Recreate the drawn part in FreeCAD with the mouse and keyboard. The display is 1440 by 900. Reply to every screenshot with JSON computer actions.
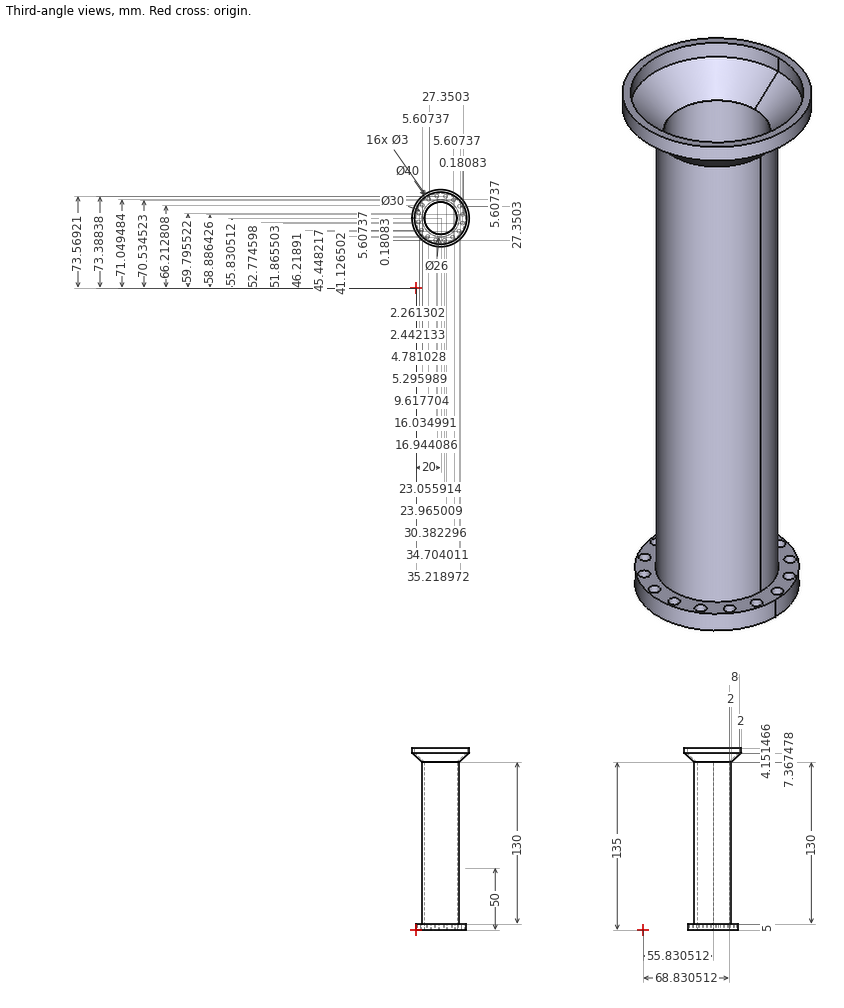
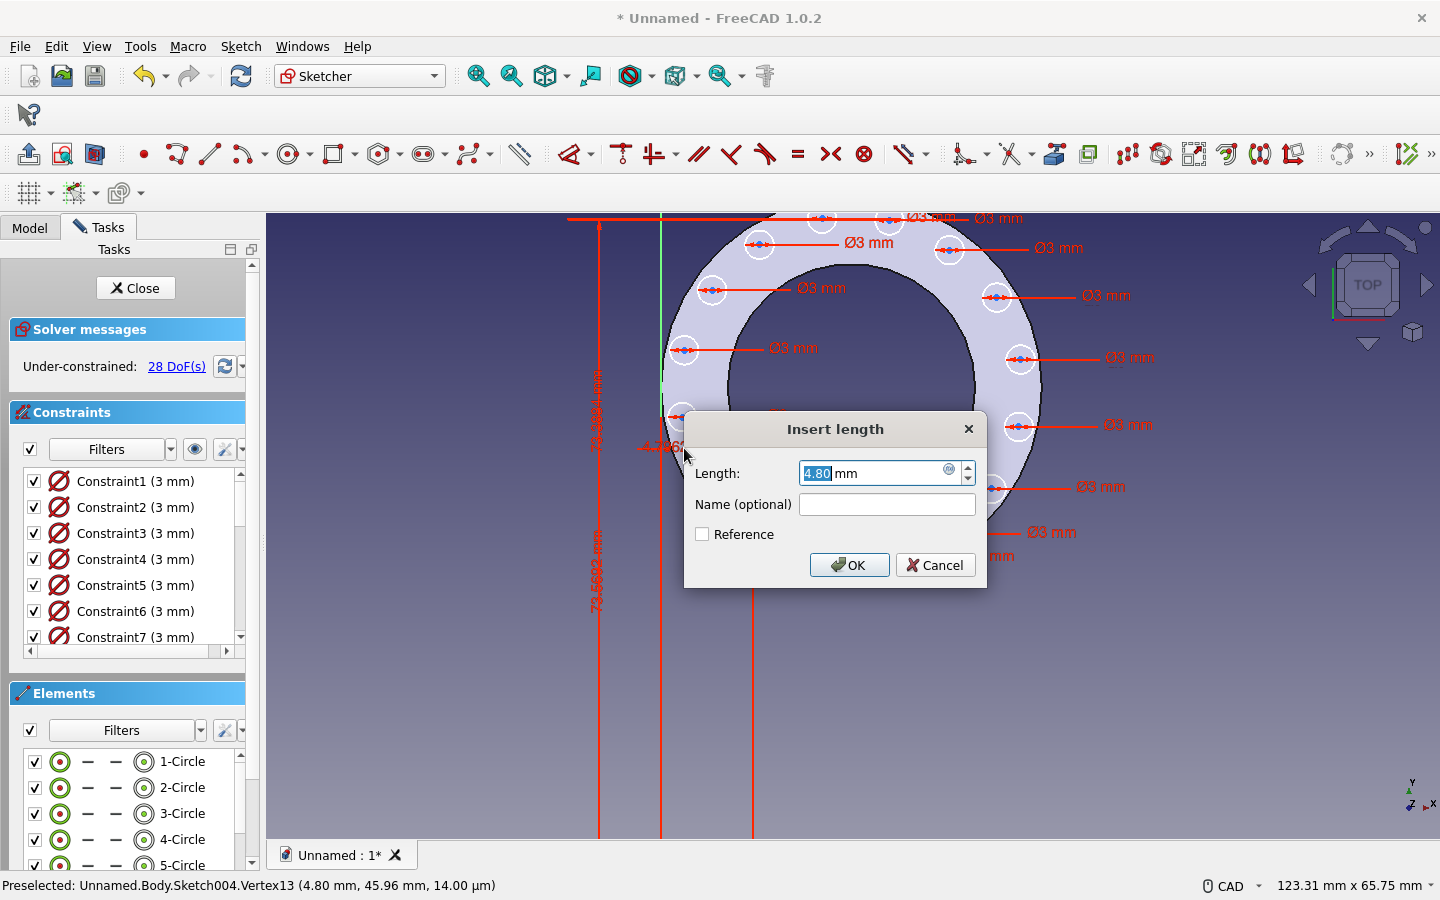
{"action": "type", "text": "4.781028"}
{"action": "key", "text": "Return"}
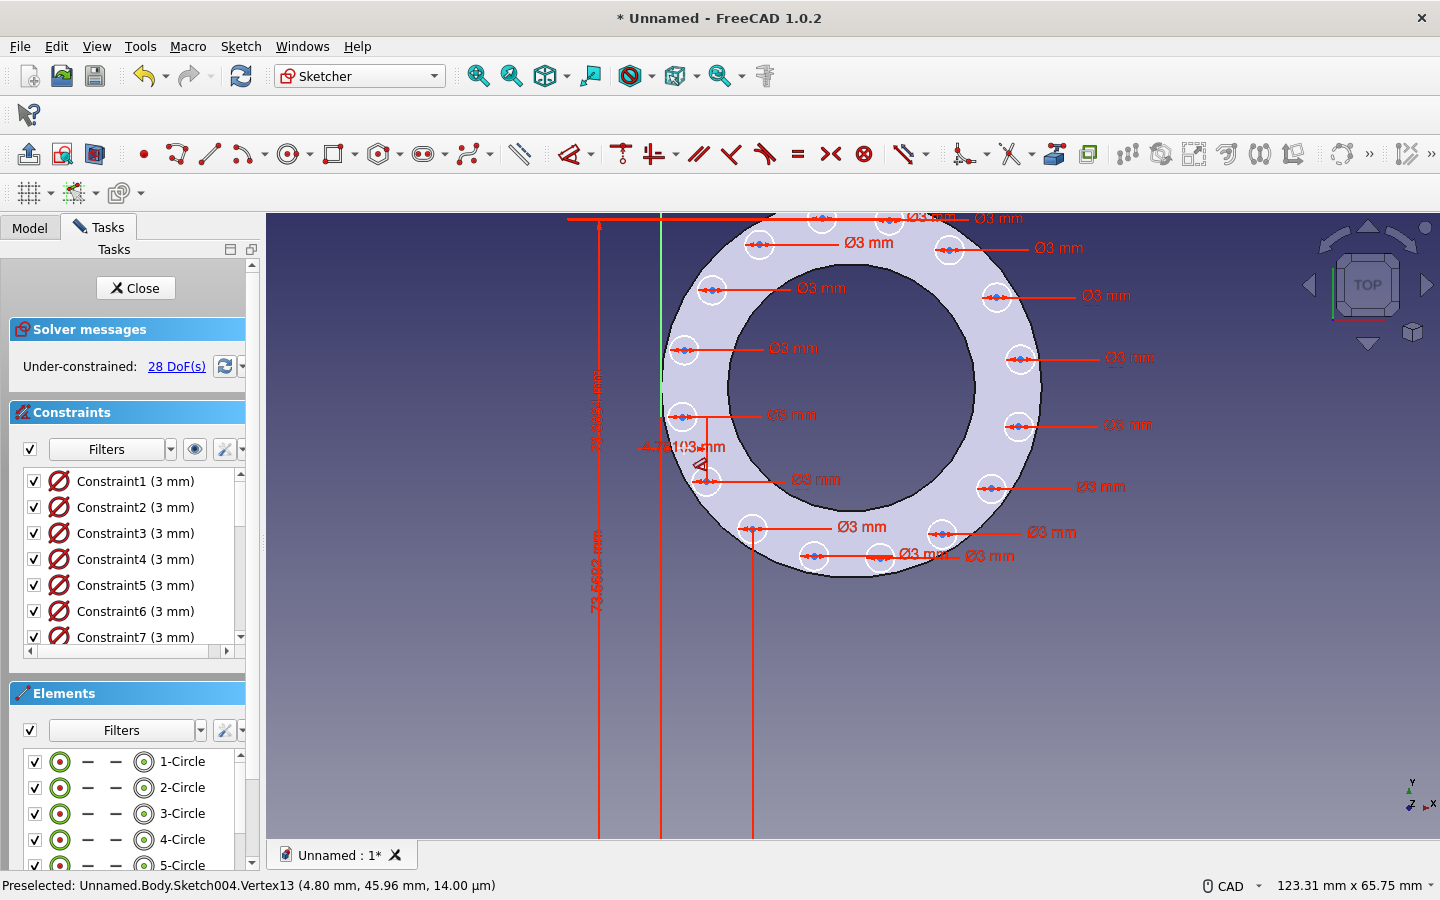
{"action": "left_click", "coordinate": [707, 482]}
{"action": "left_click", "coordinate": [627, 646]}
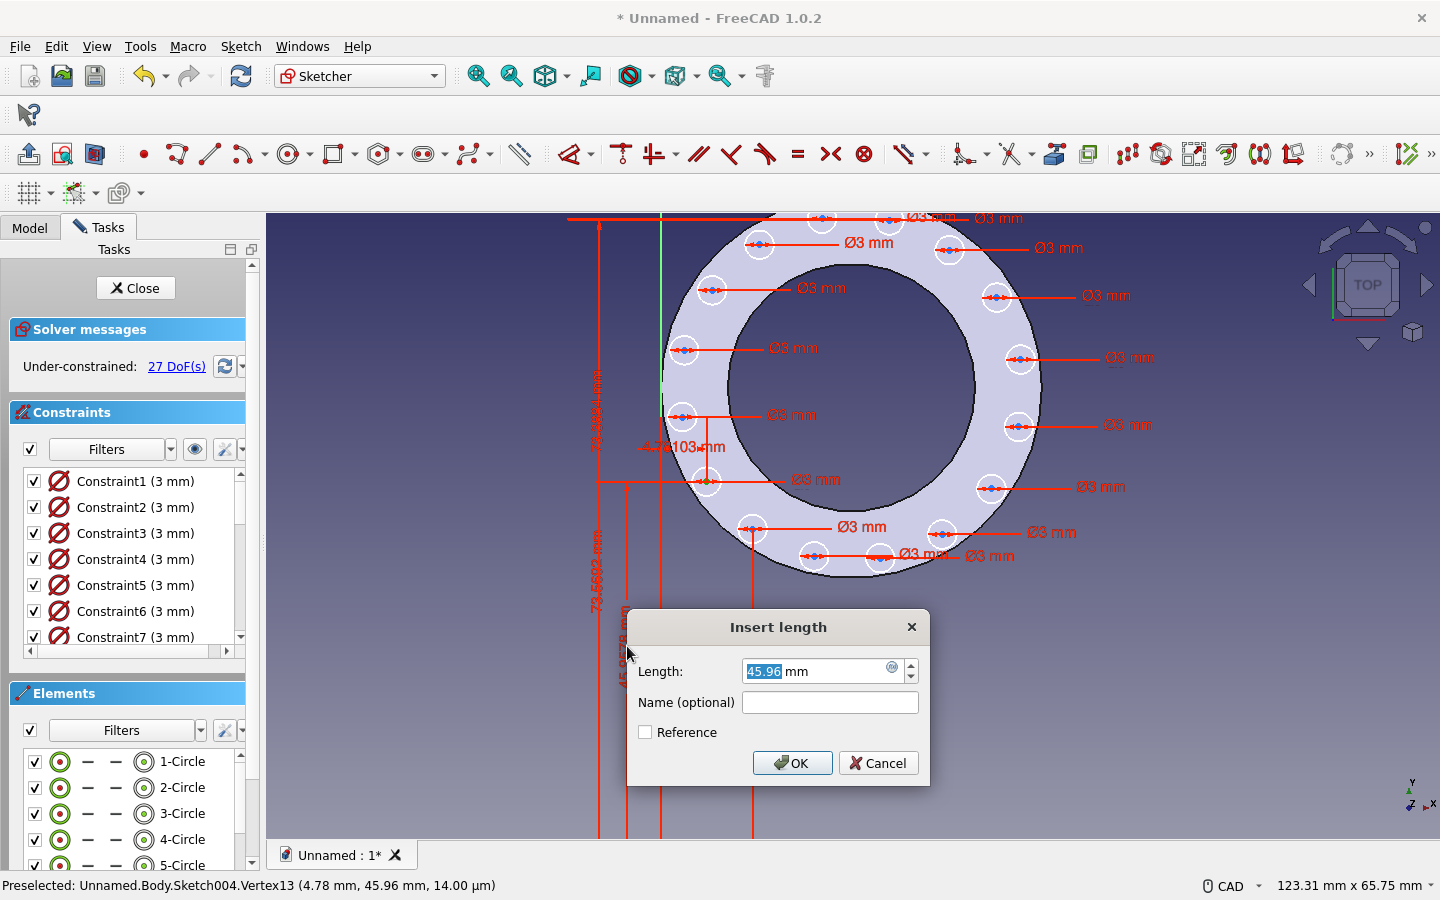
{"action": "type", "text": "46.21891"}
{"action": "key", "text": "Return"}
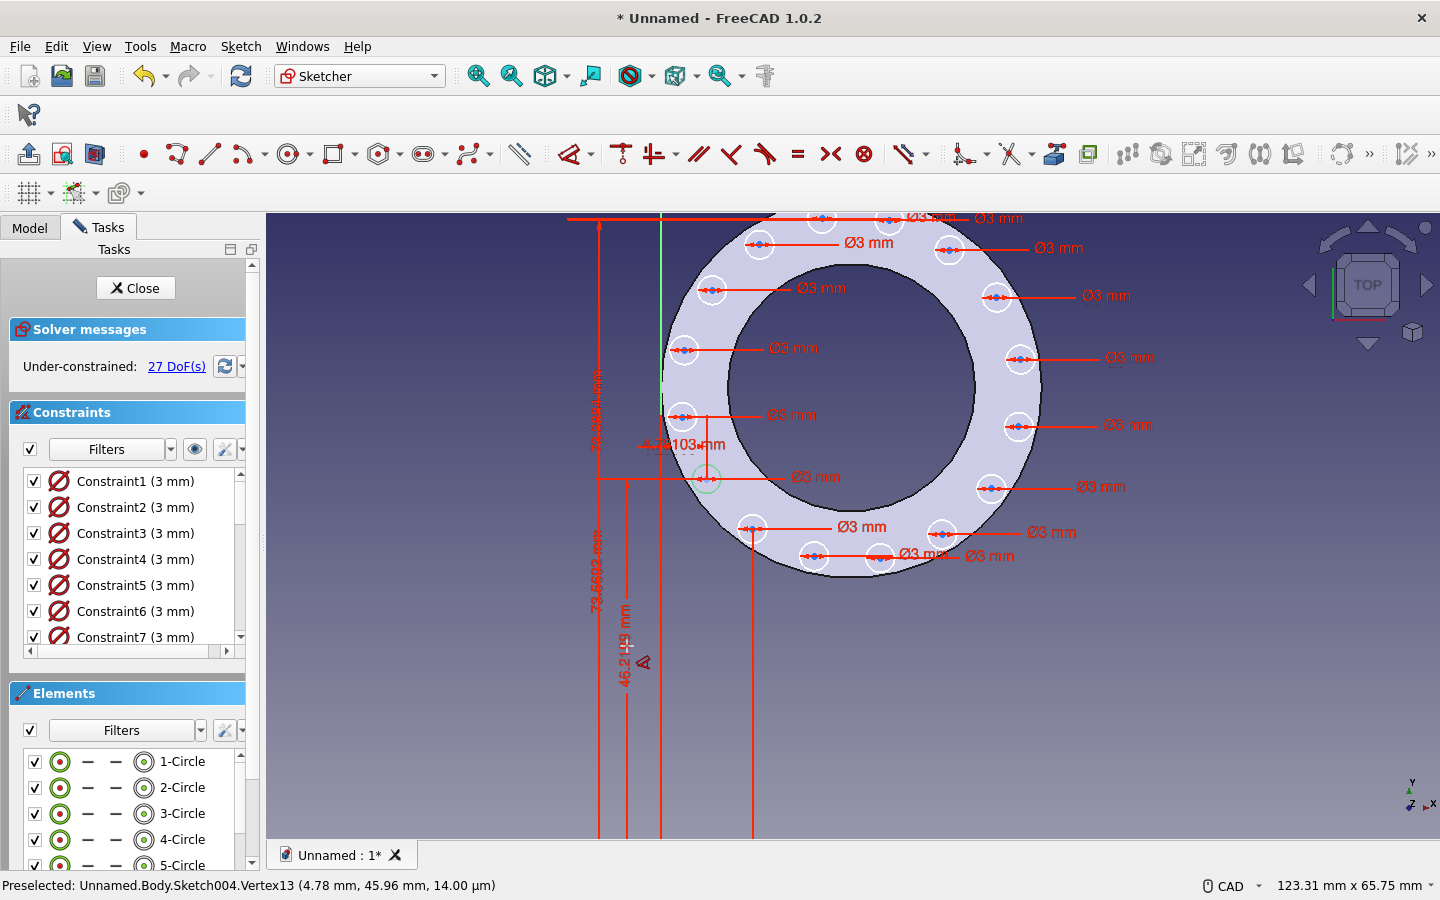
{"action": "scroll", "coordinate": [682, 417], "scroll_direction": "up", "scroll_amount": 4}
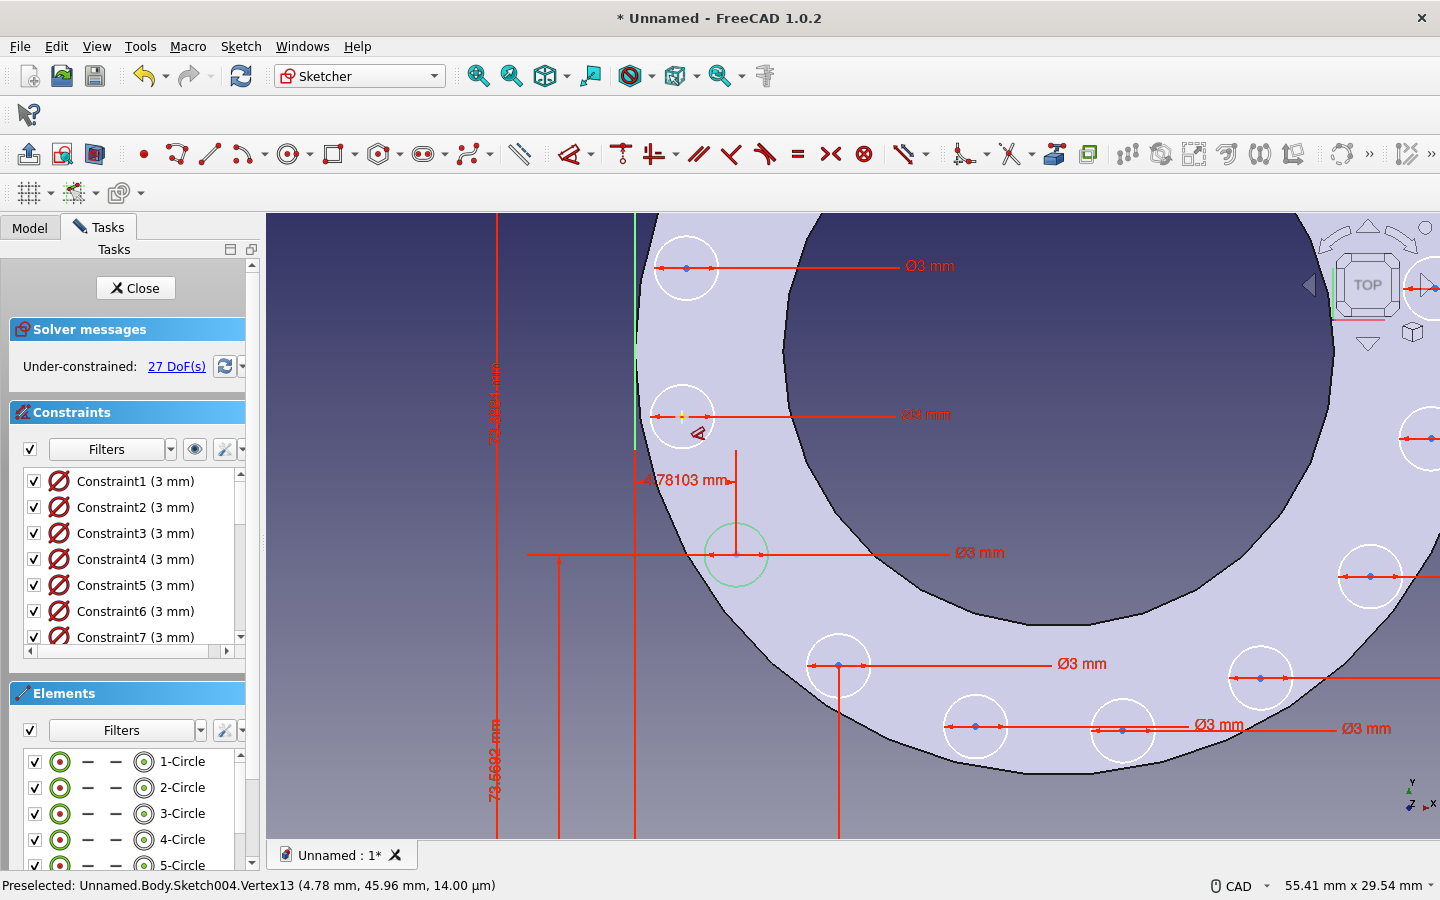
{"action": "left_click", "coordinate": [682, 417]}
{"action": "left_click", "coordinate": [659, 359]}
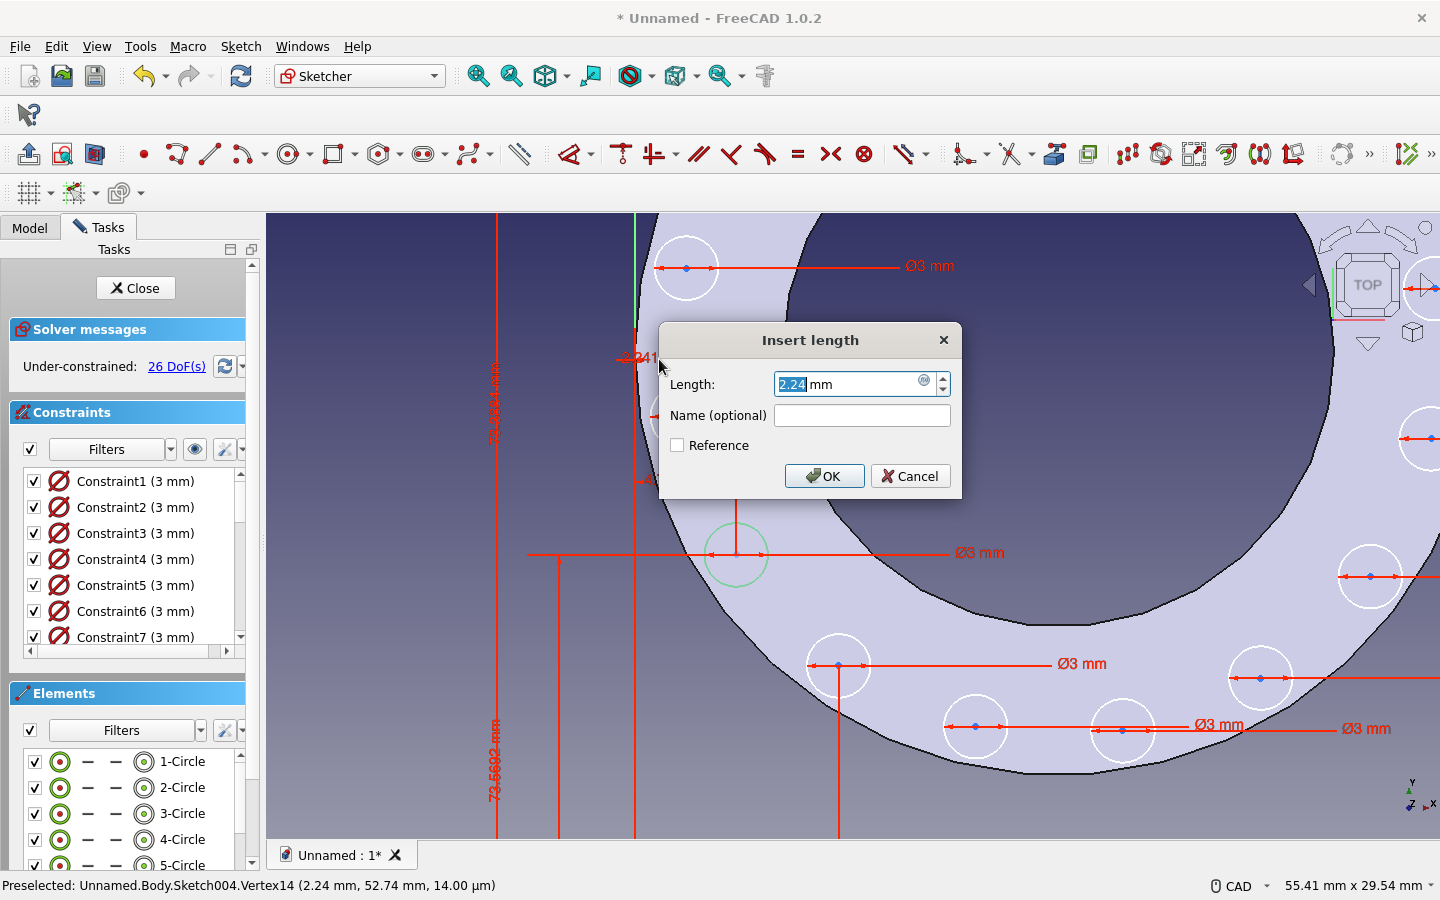
{"action": "type", "text": "2.261302"}
{"action": "key", "text": "Return"}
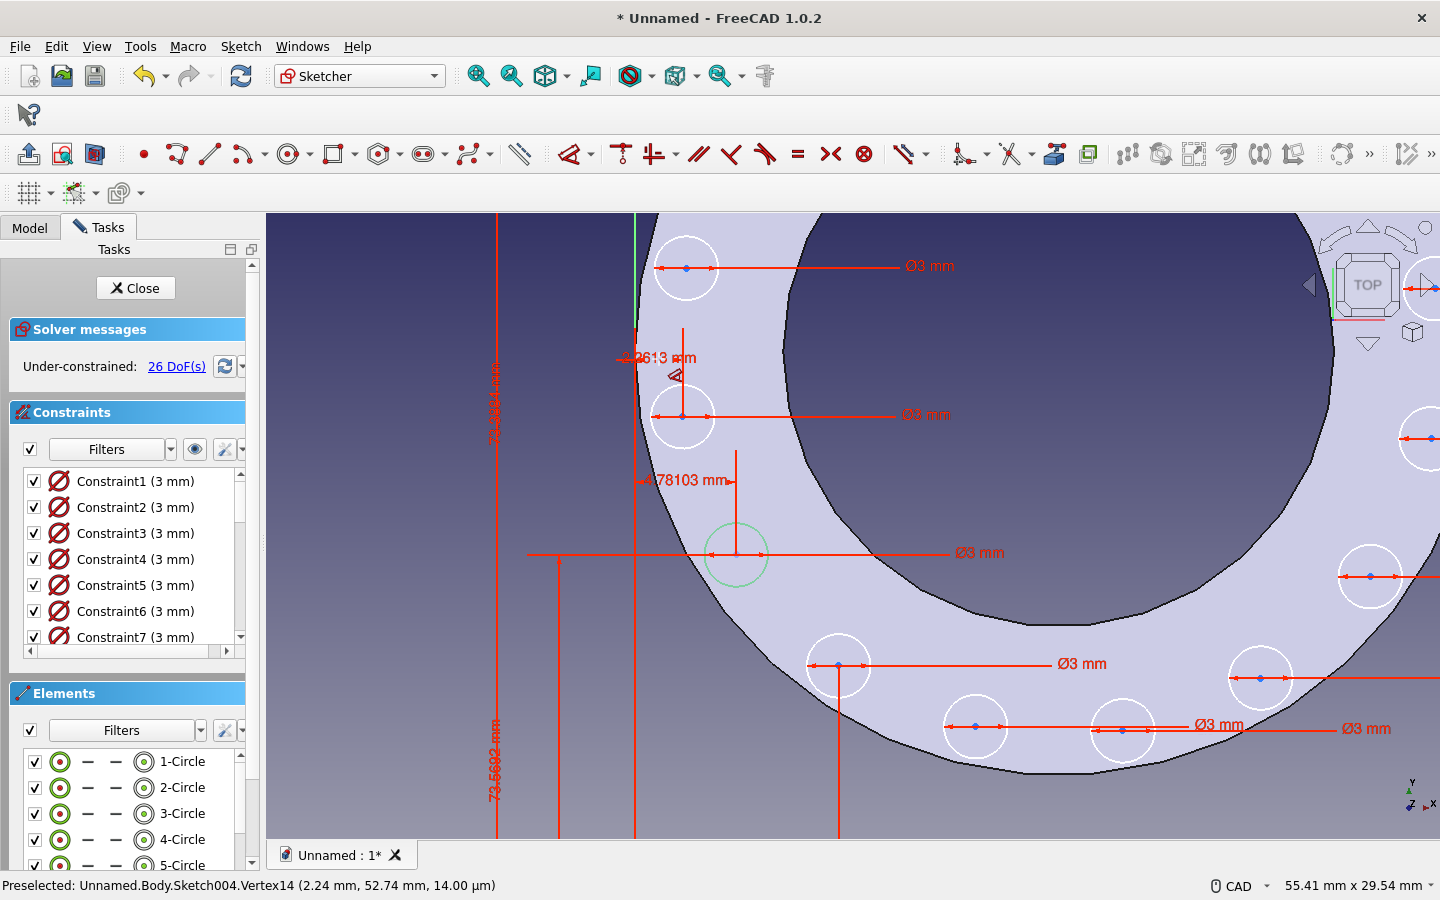
{"action": "left_click", "coordinate": [686, 268]}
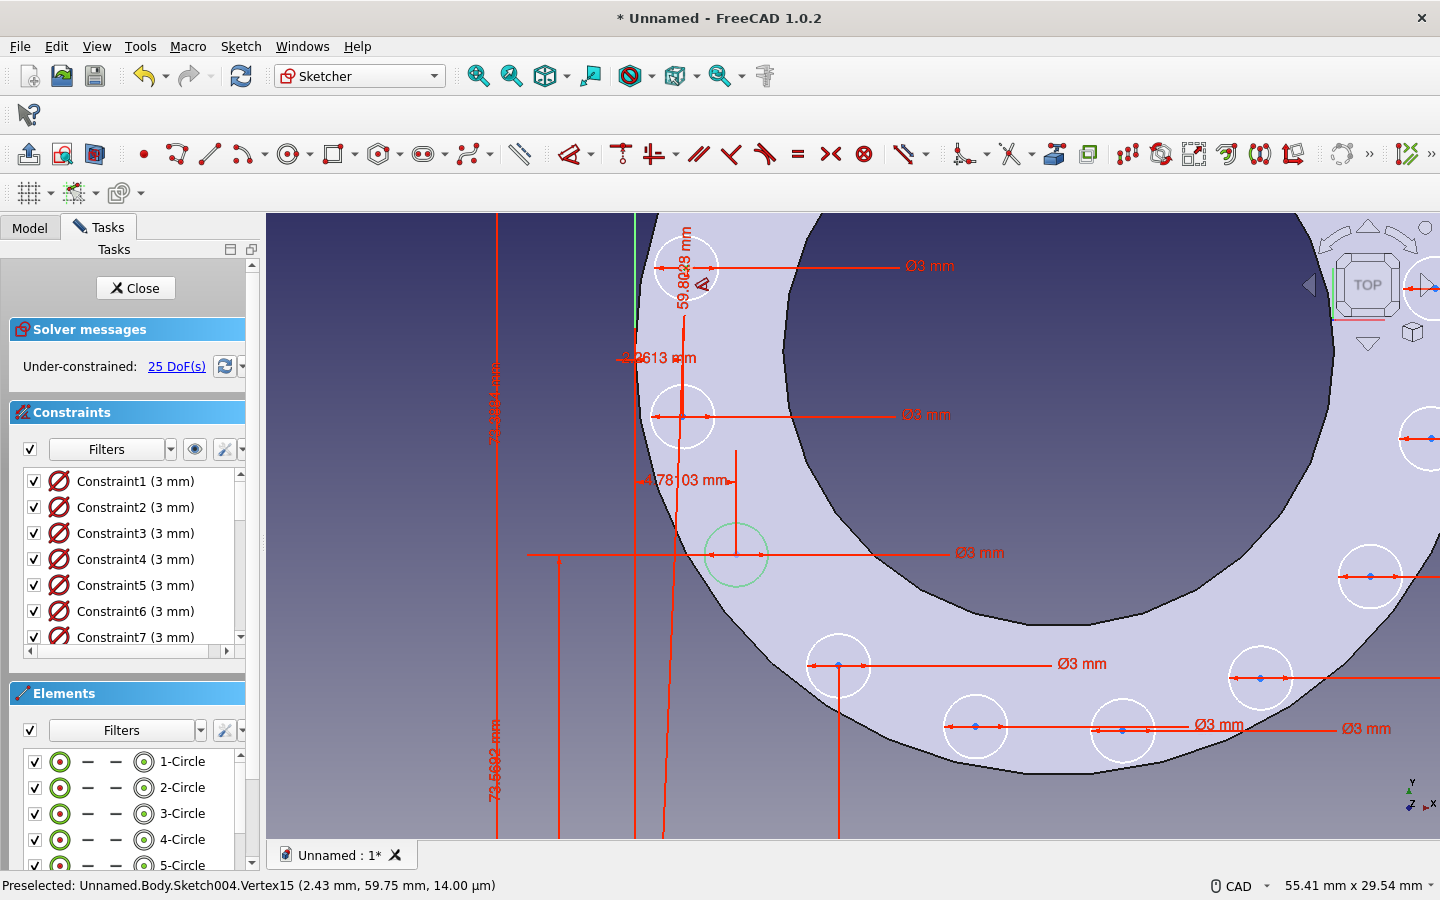
{"action": "key", "text": "Escape"}
{"action": "key", "text": "Escape"}